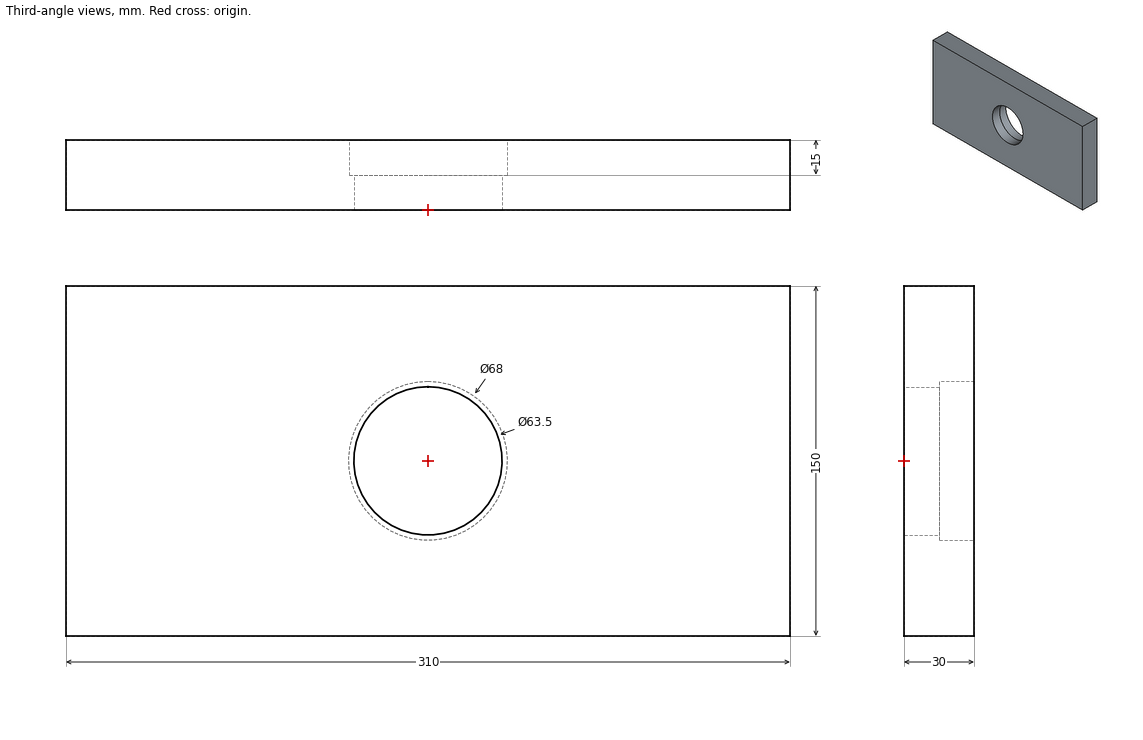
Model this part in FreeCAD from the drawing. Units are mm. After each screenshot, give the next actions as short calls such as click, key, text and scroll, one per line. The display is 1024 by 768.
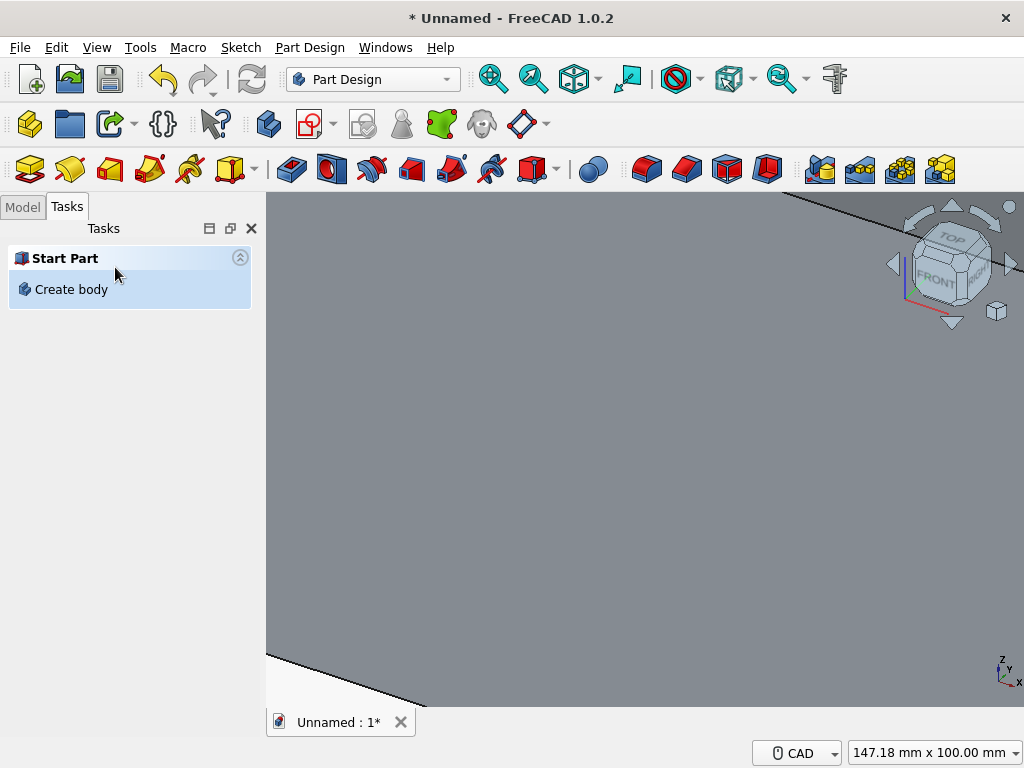
click(494, 80)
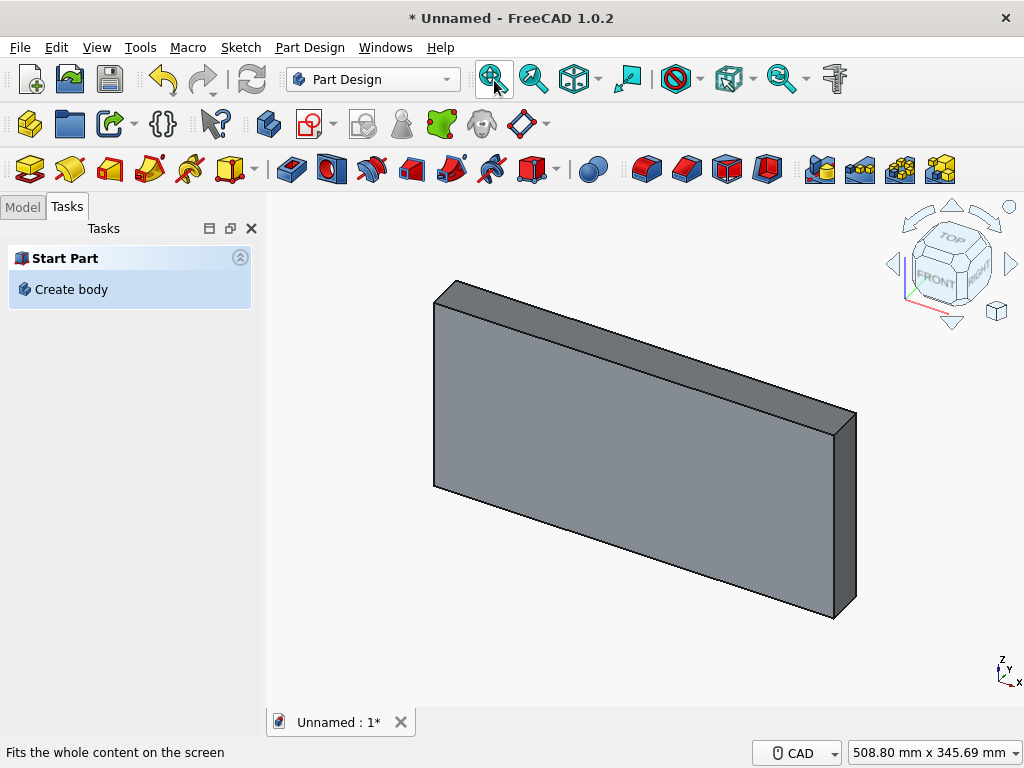
key(4)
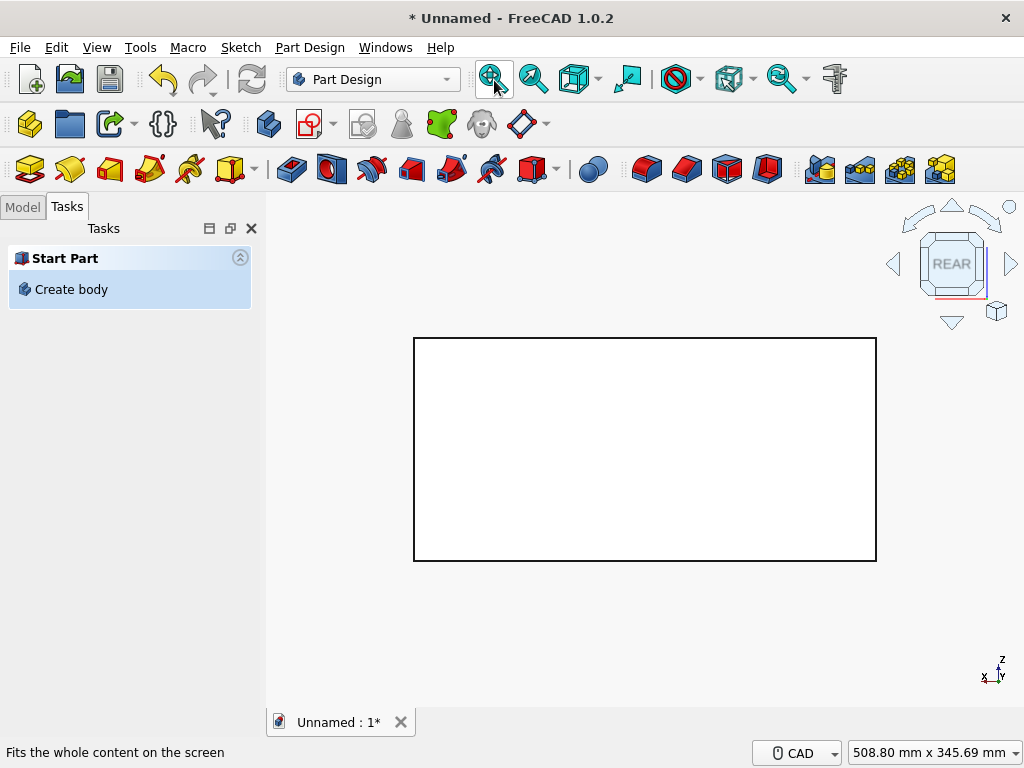
click(579, 448)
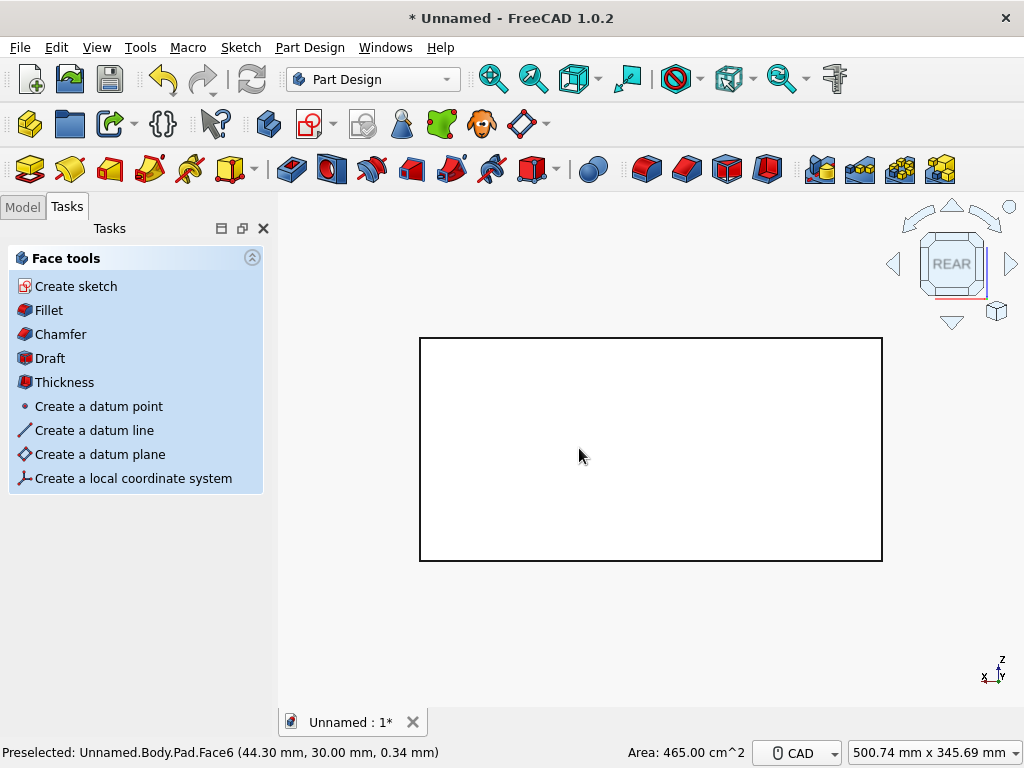
click(310, 124)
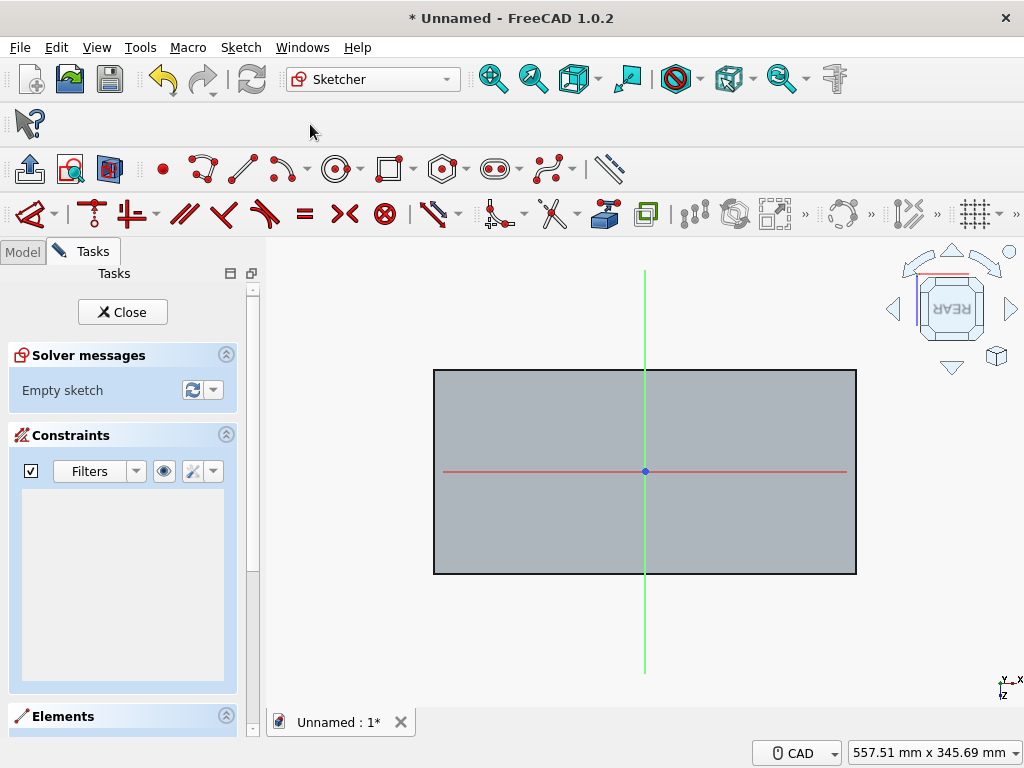
scroll(675, 472, up, 6)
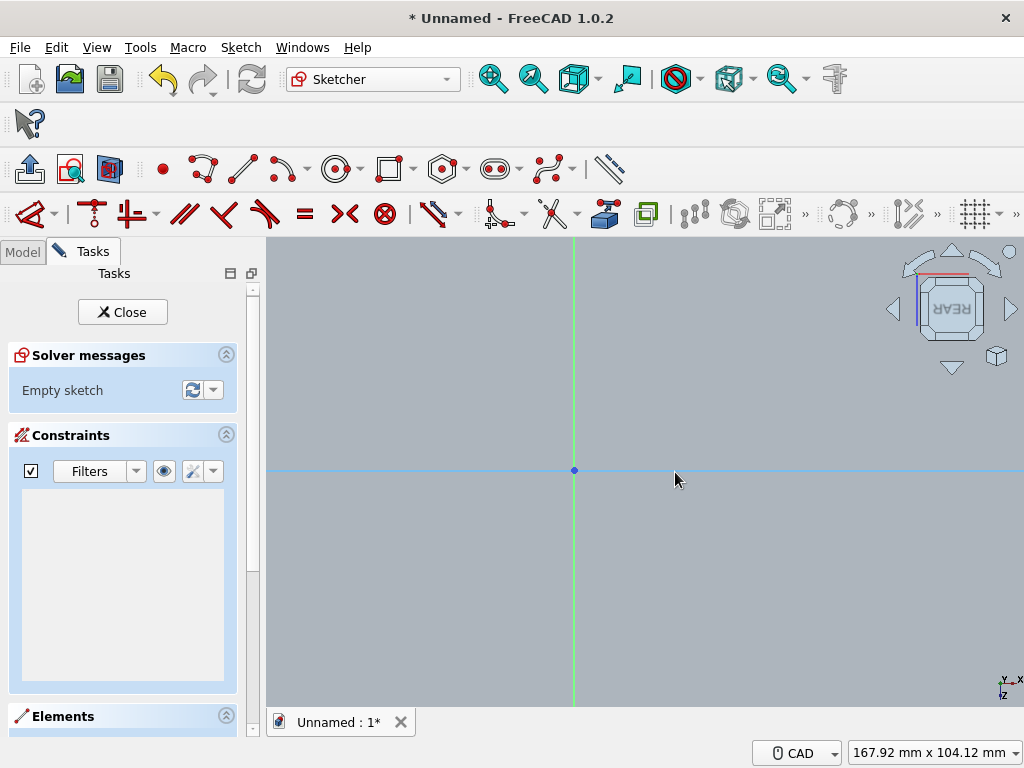
click(336, 170)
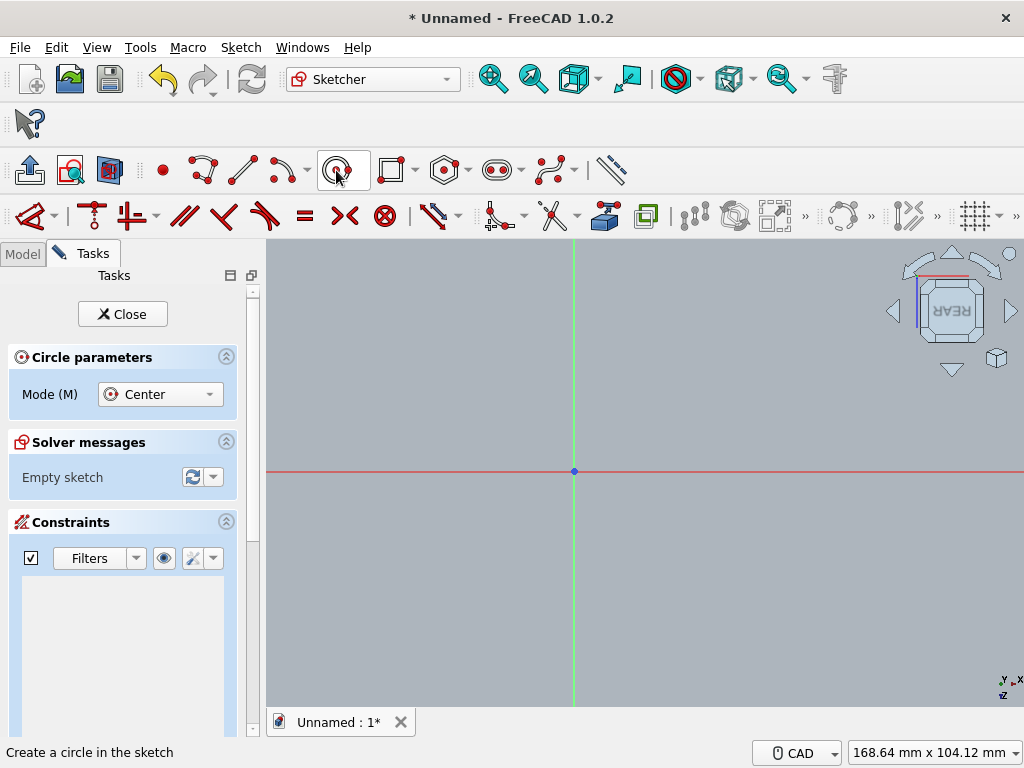
click(574, 472)
move(675, 371)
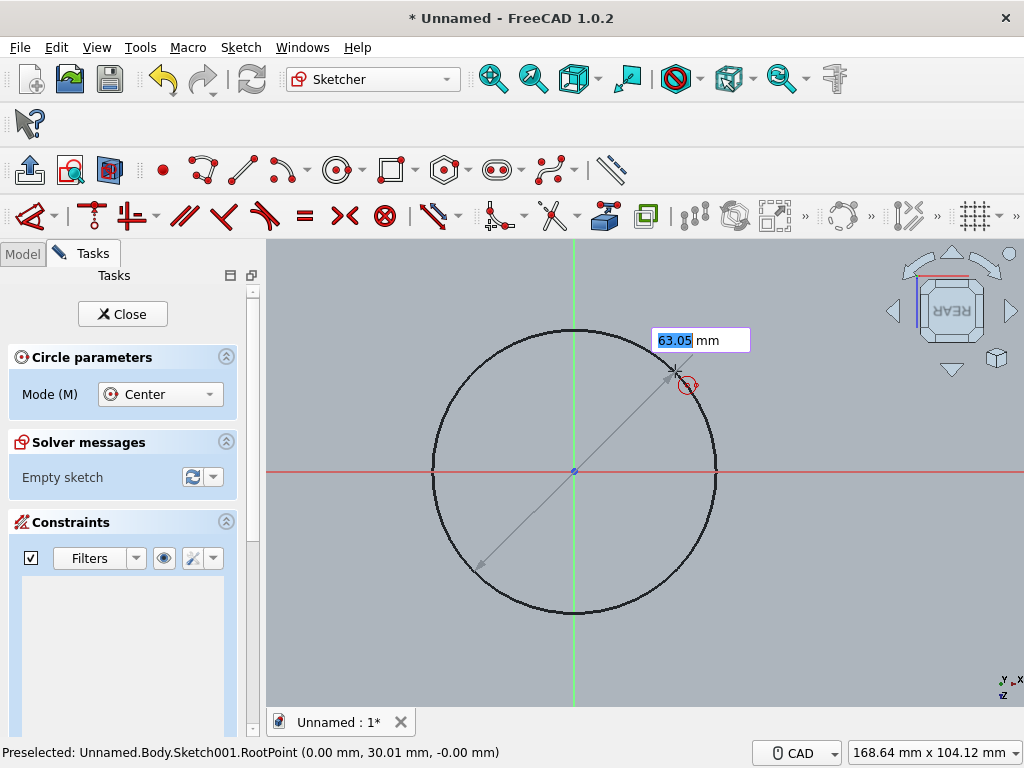
text(63.5)
key(Return)
key(Escape)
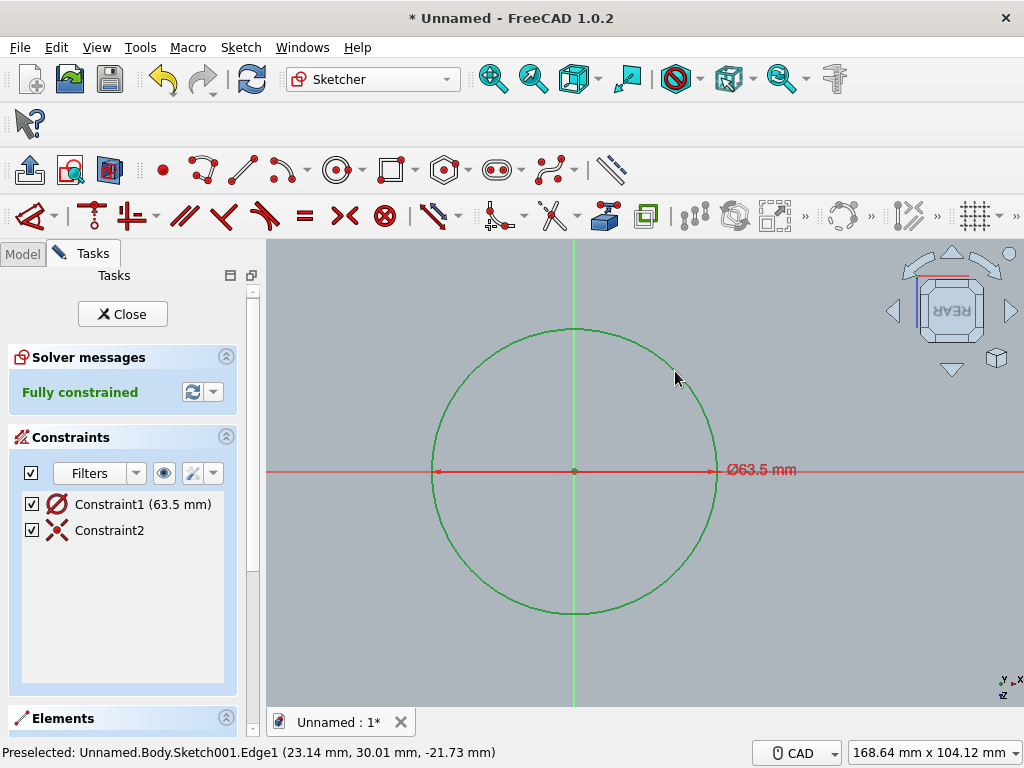
click(123, 314)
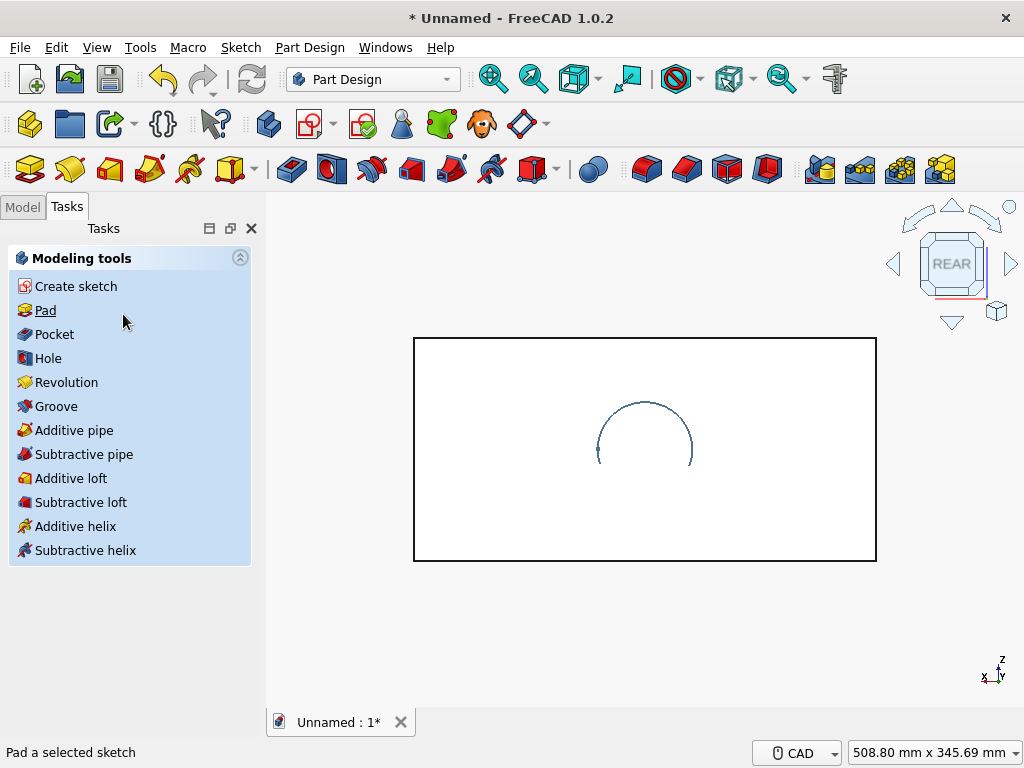
click(292, 170)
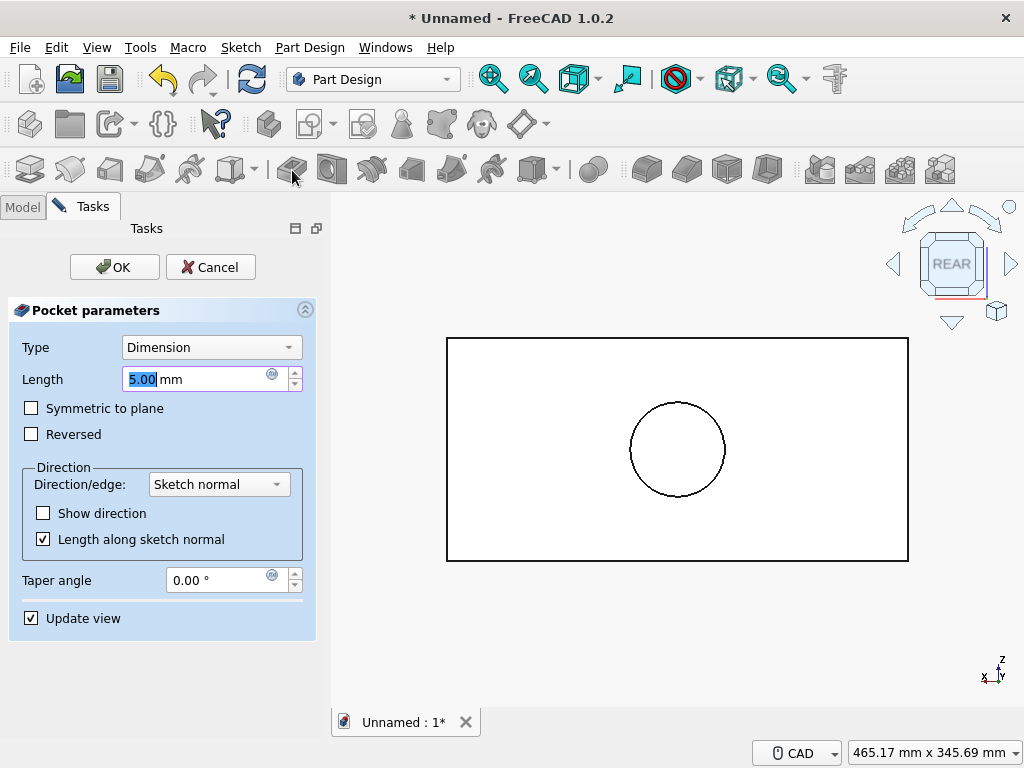
click(212, 348)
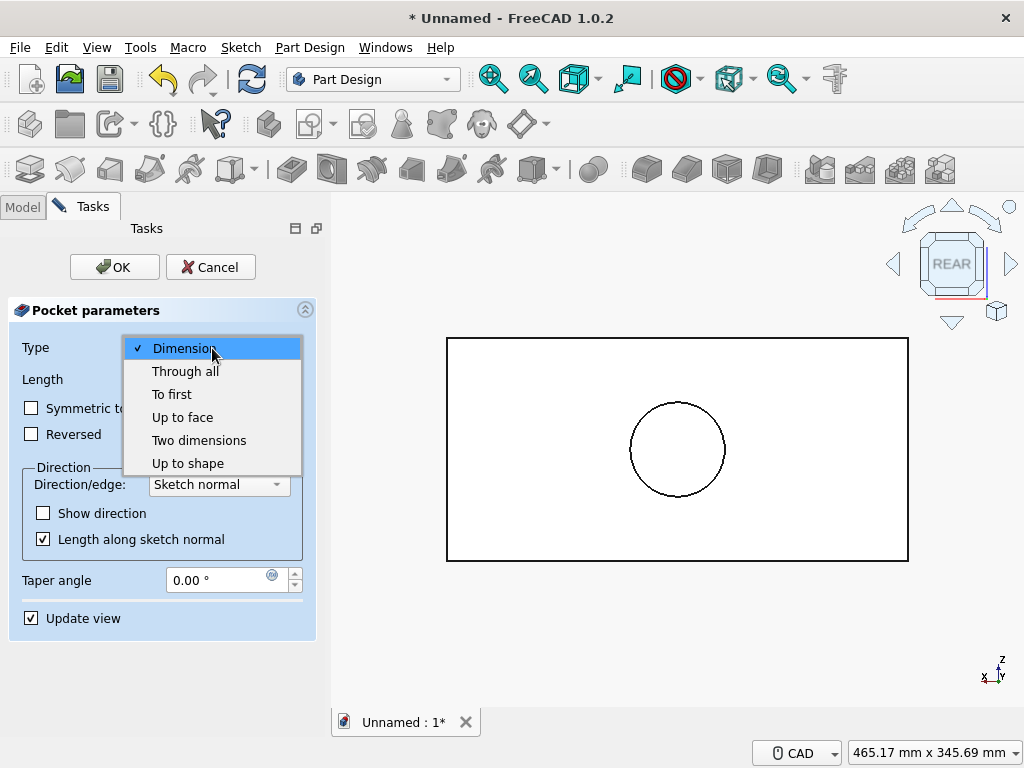
click(212, 372)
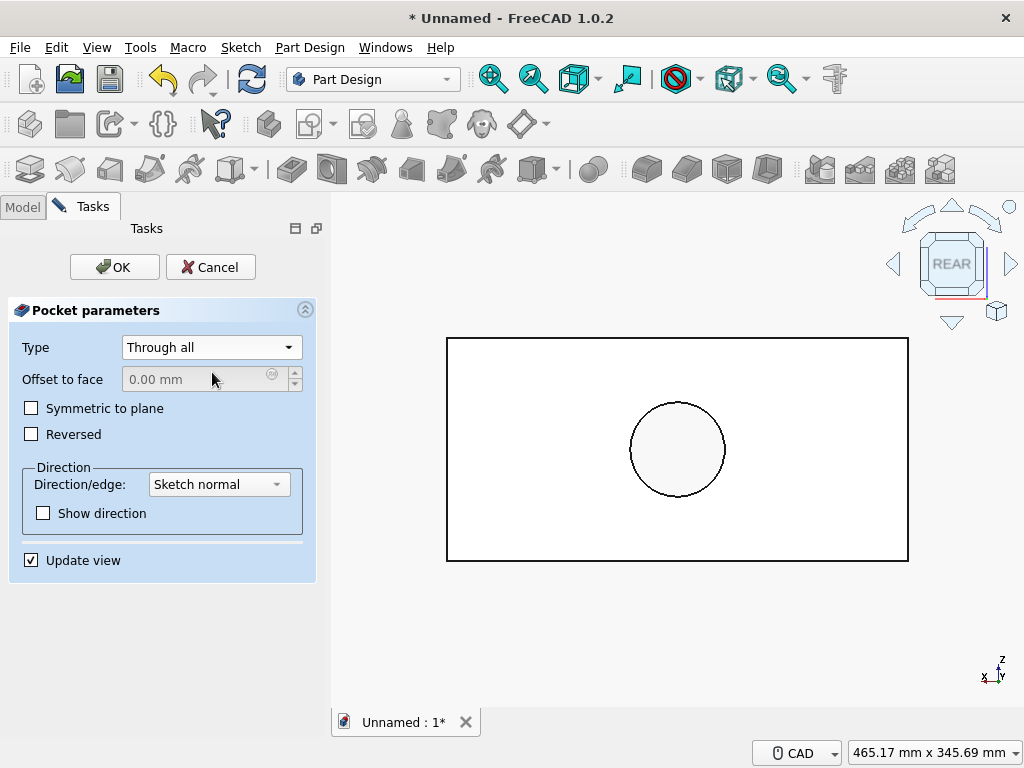
click(115, 267)